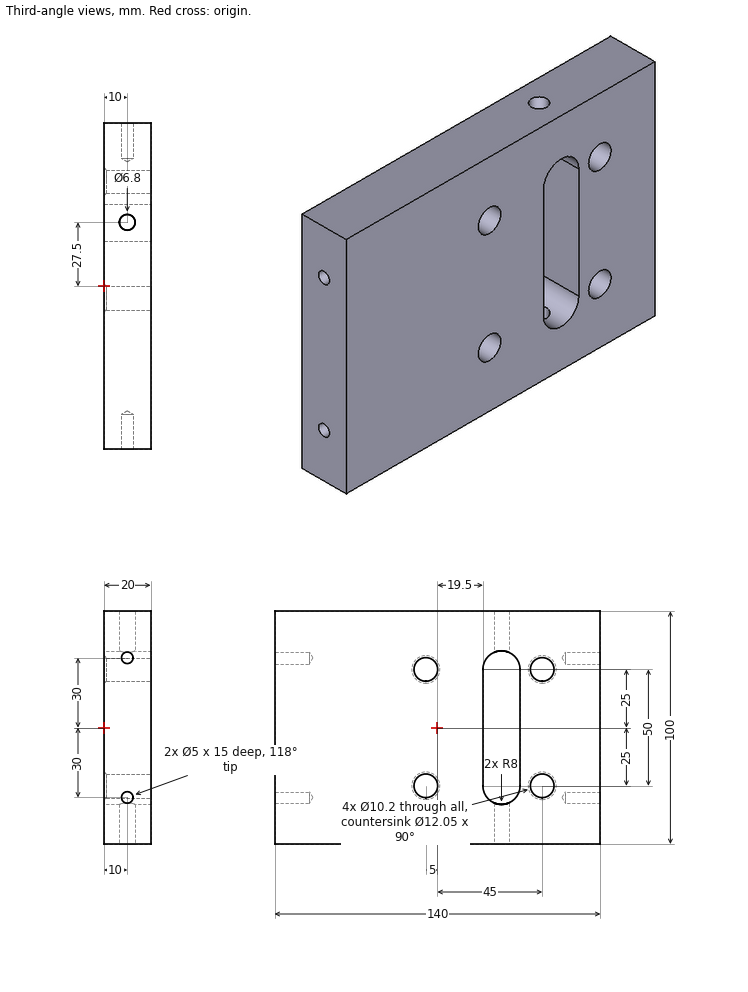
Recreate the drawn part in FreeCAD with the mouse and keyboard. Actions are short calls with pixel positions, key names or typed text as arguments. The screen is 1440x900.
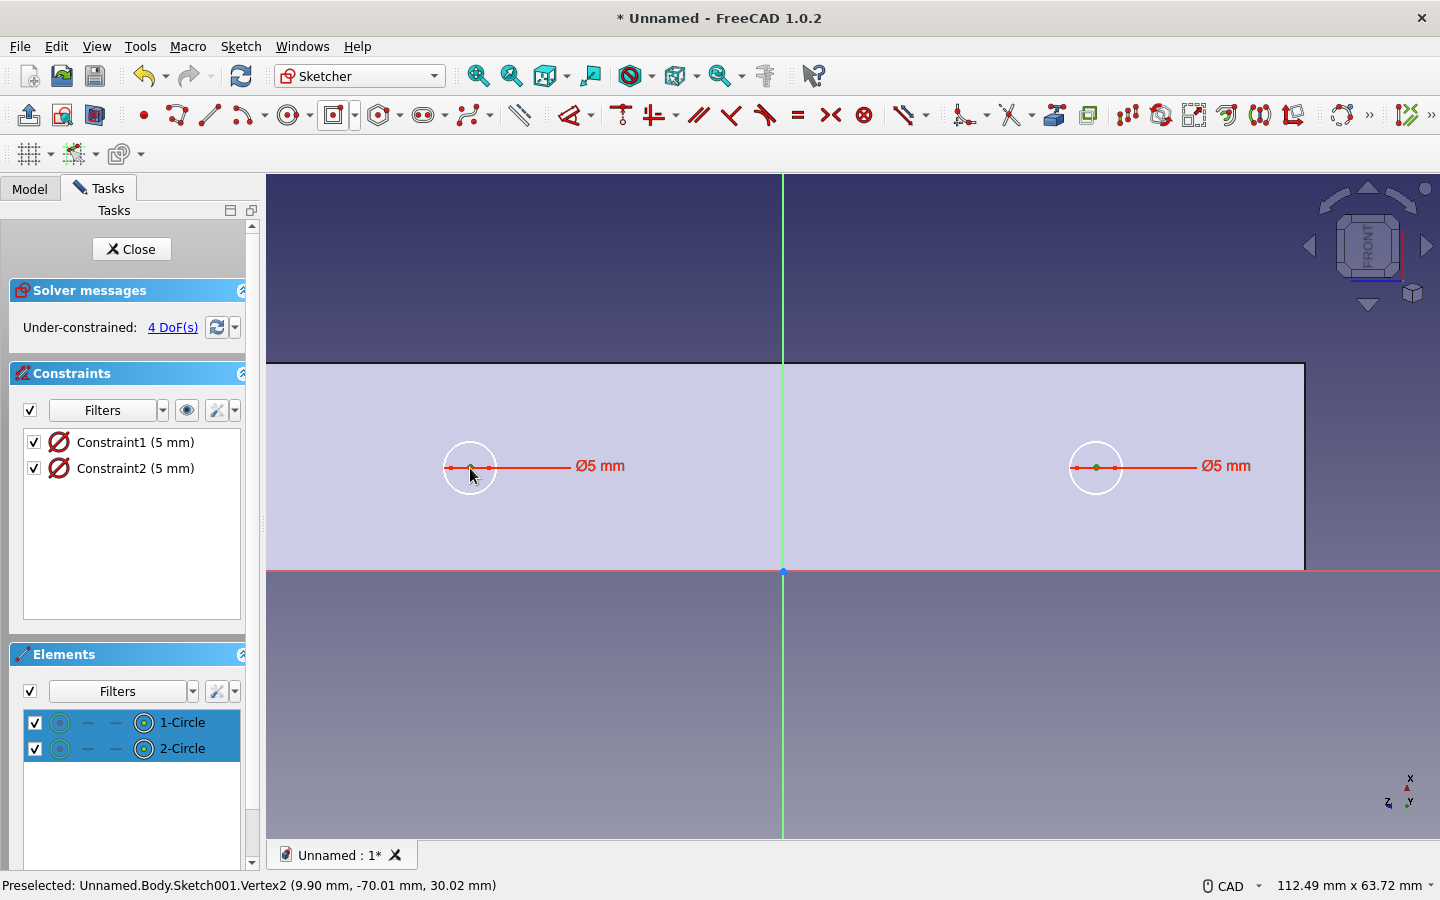
key(h)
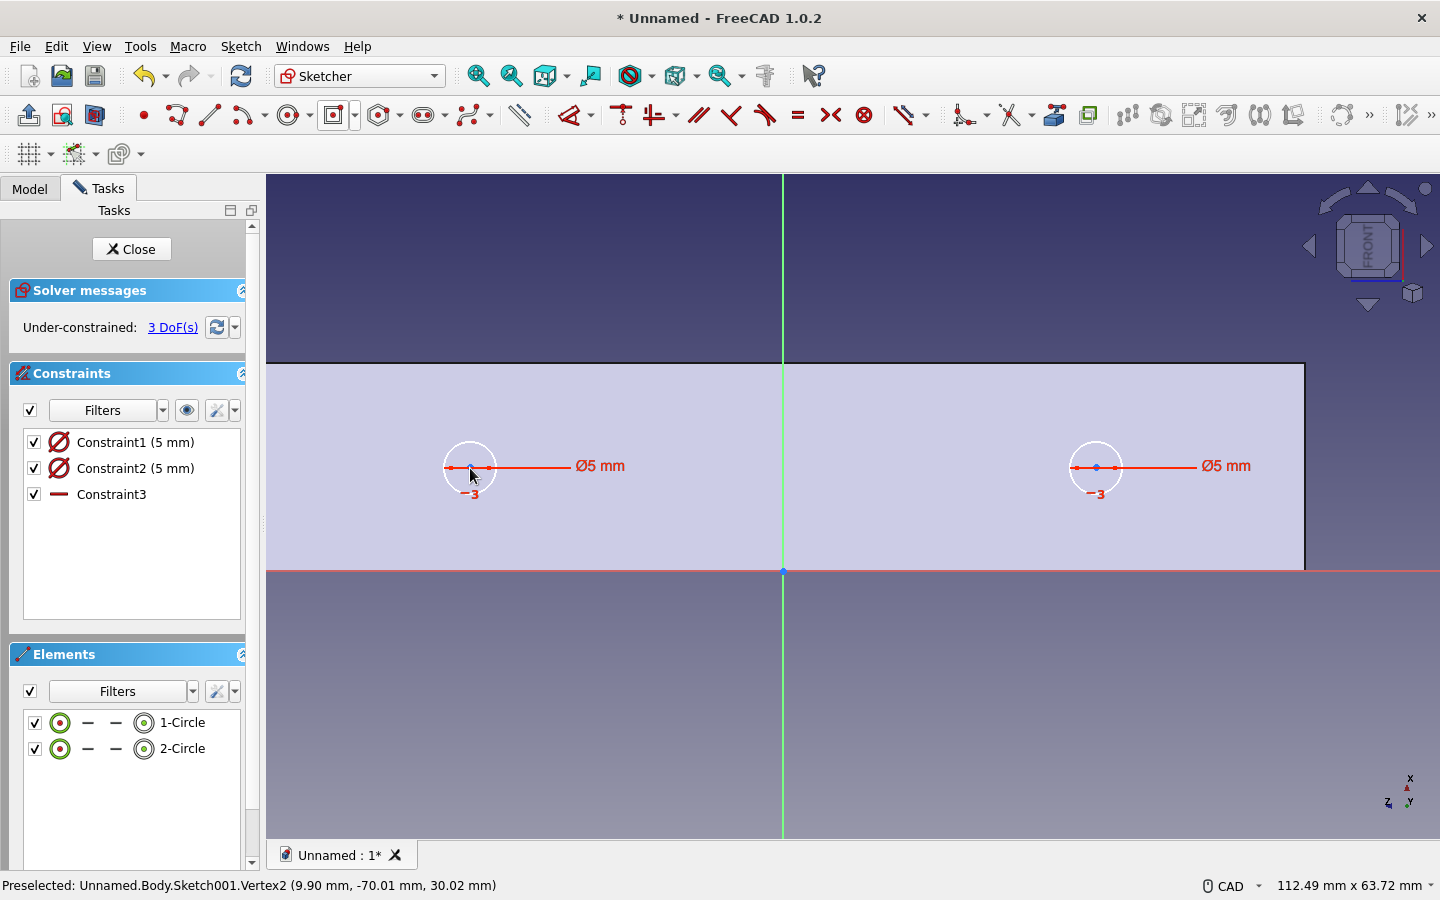
click(568, 116)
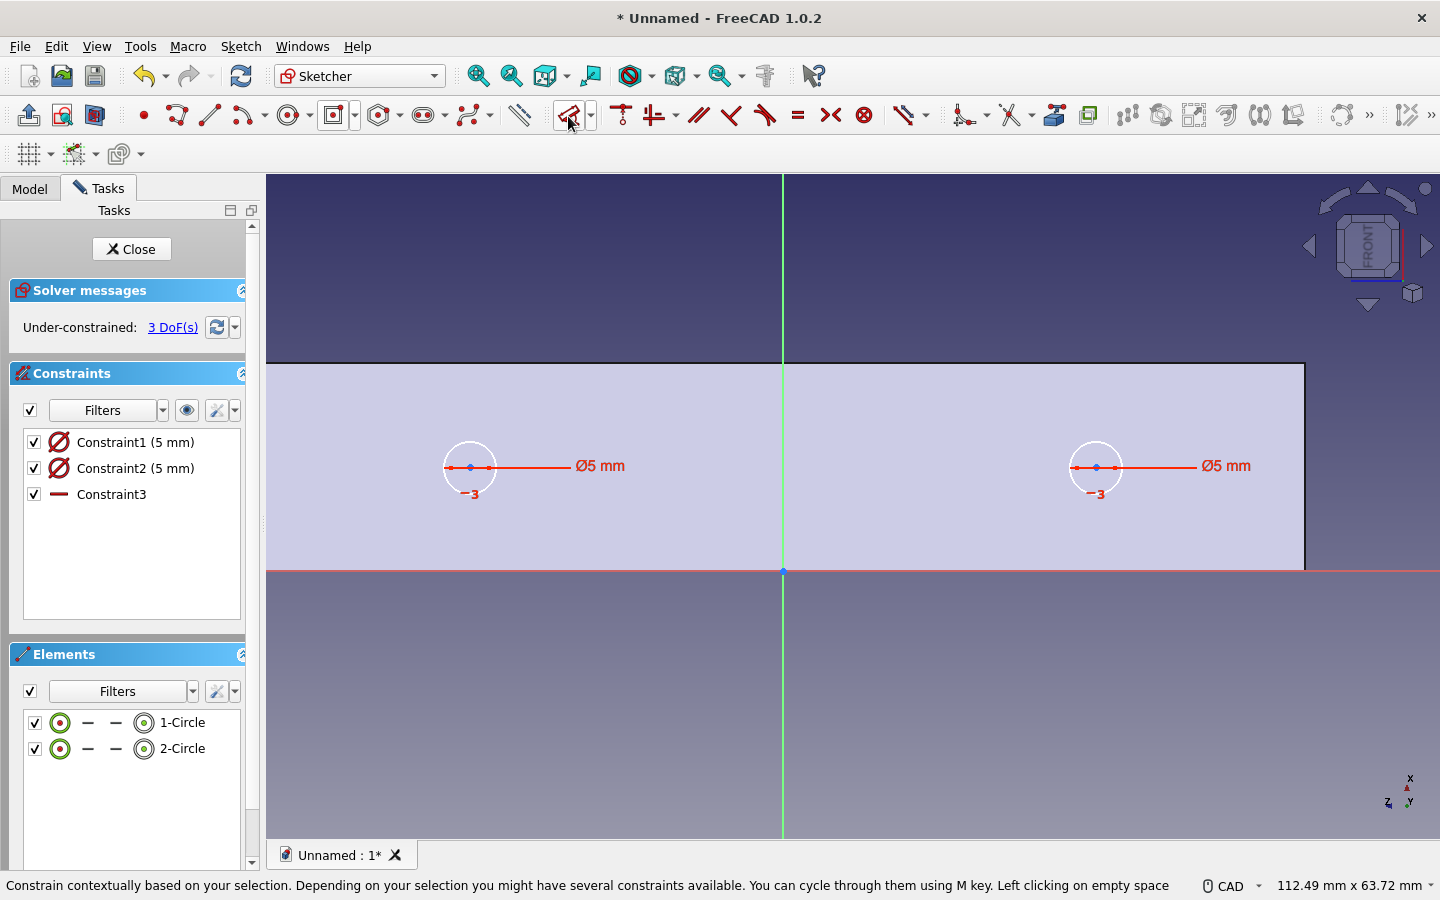
click(1096, 468)
click(940, 605)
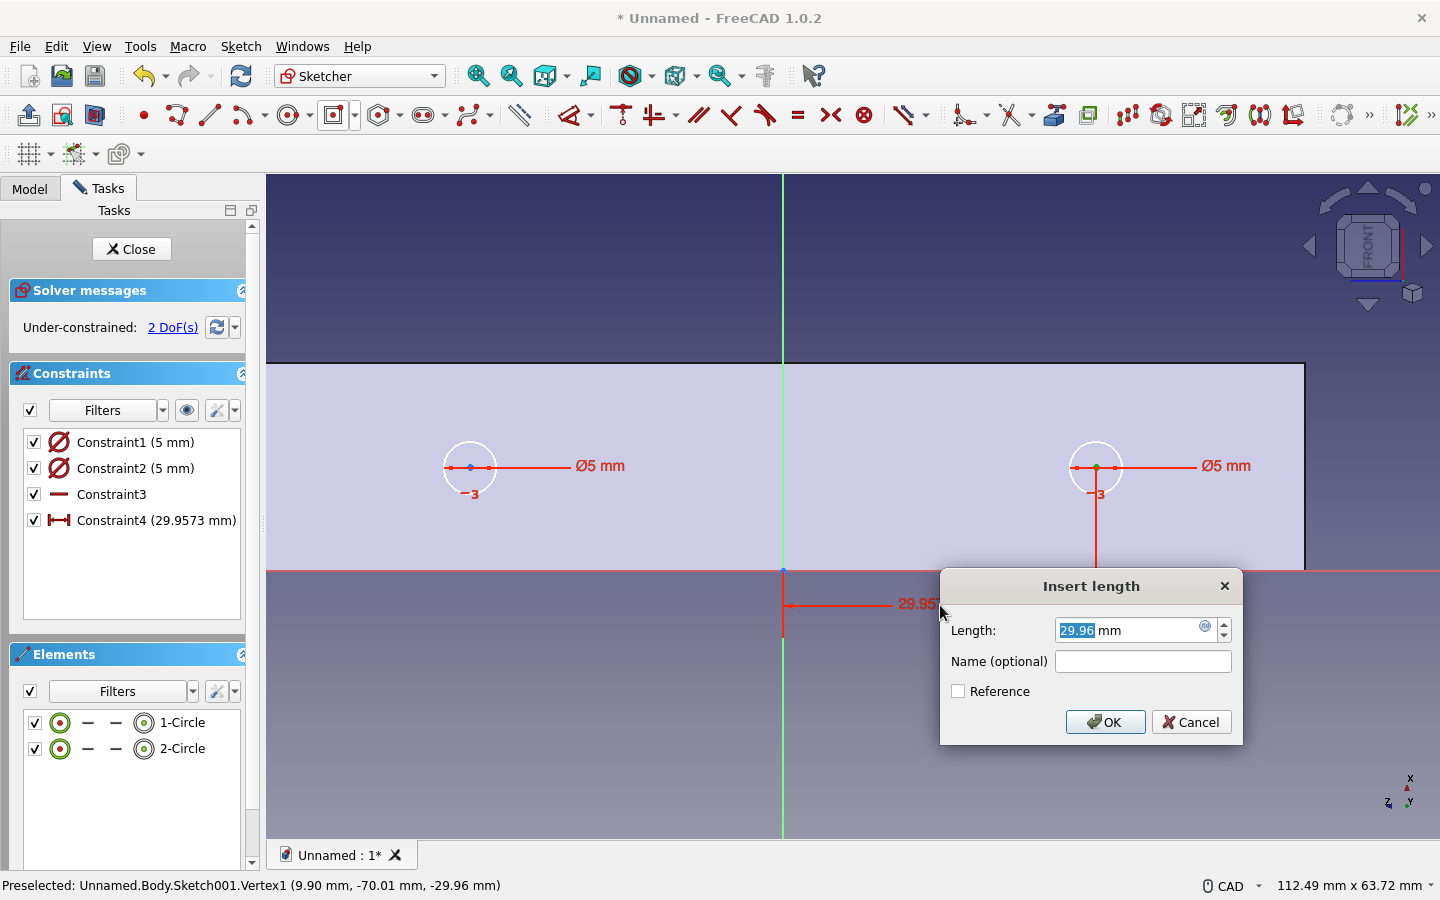
text(30)
key(Return)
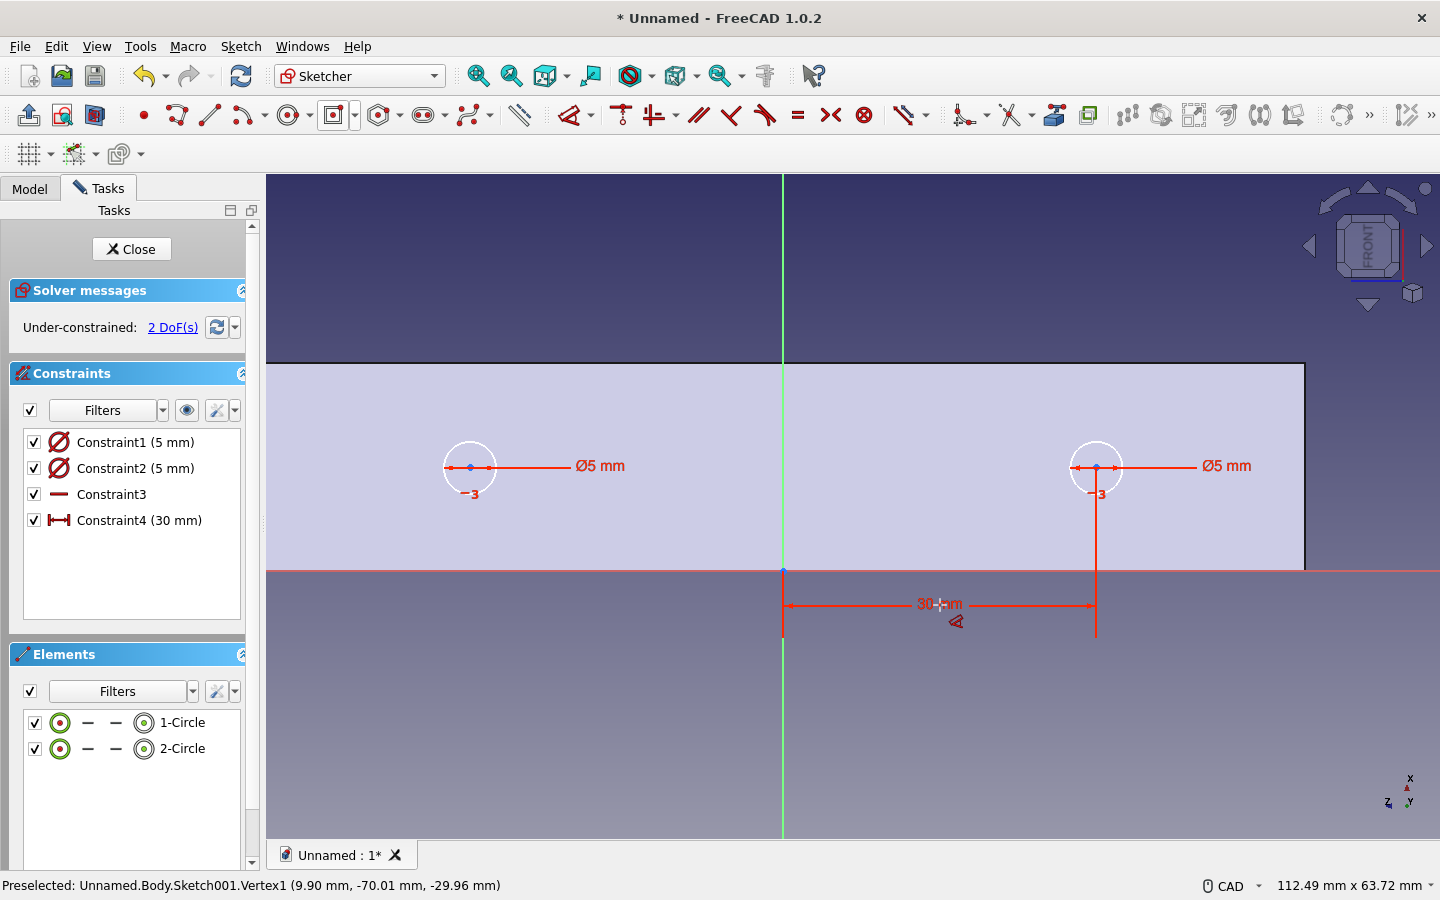
click(1096, 468)
click(1130, 520)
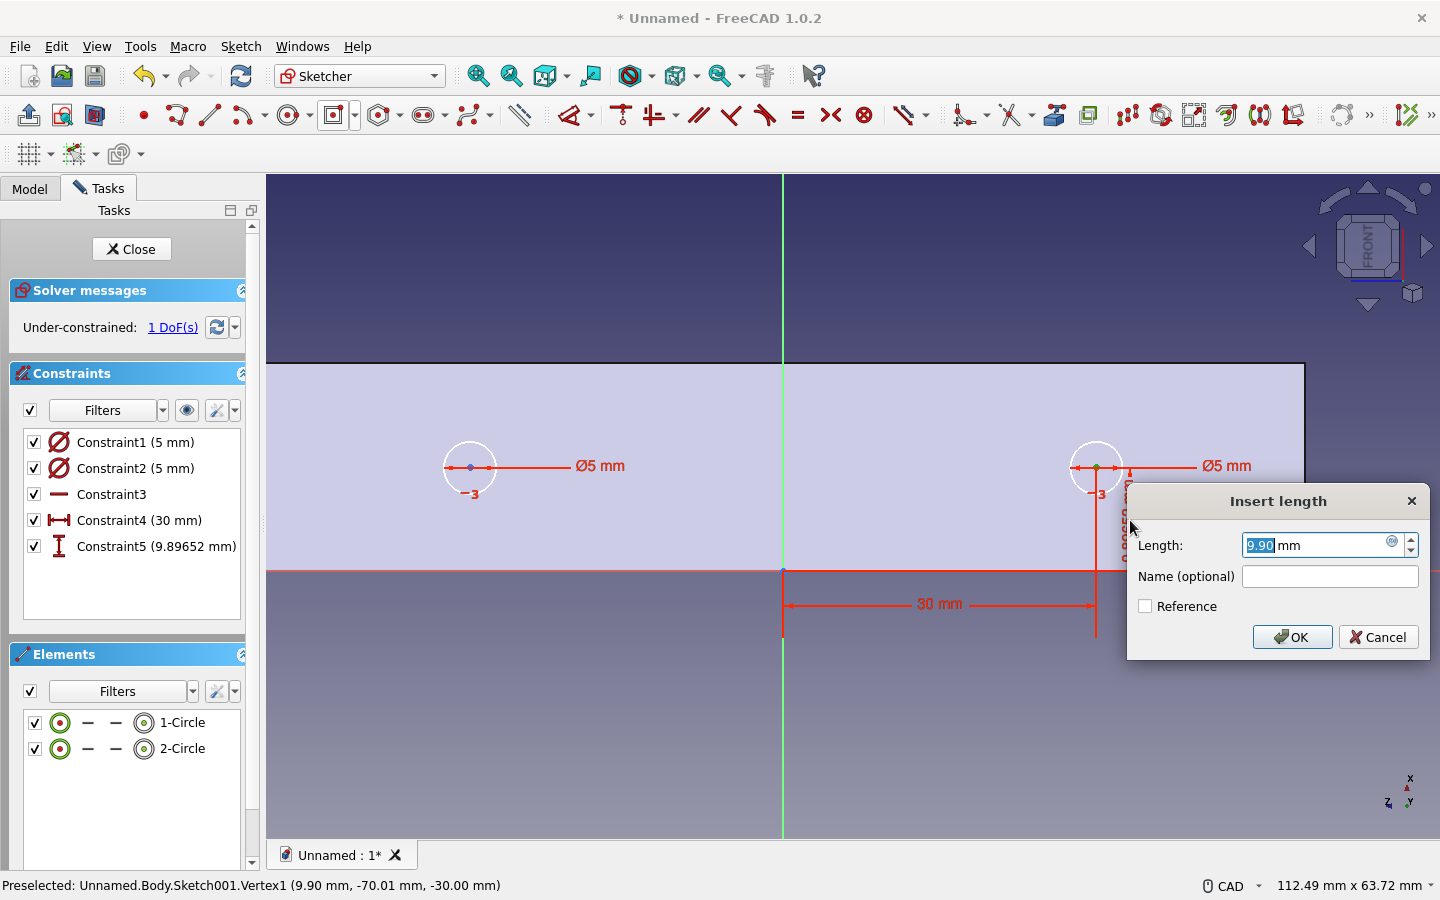
text(10)
key(Return)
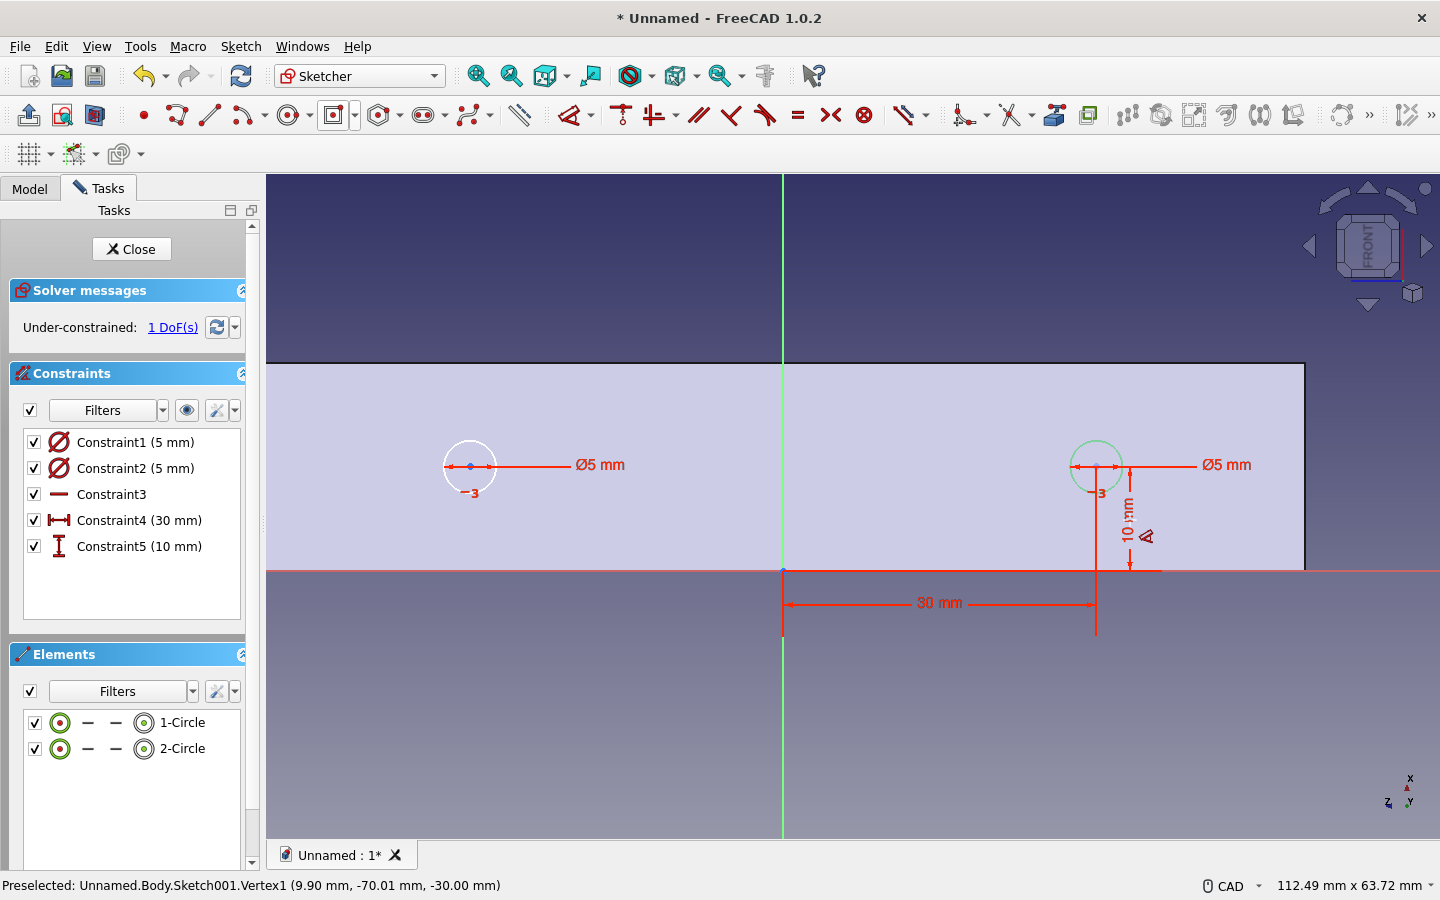
click(470, 467)
click(627, 605)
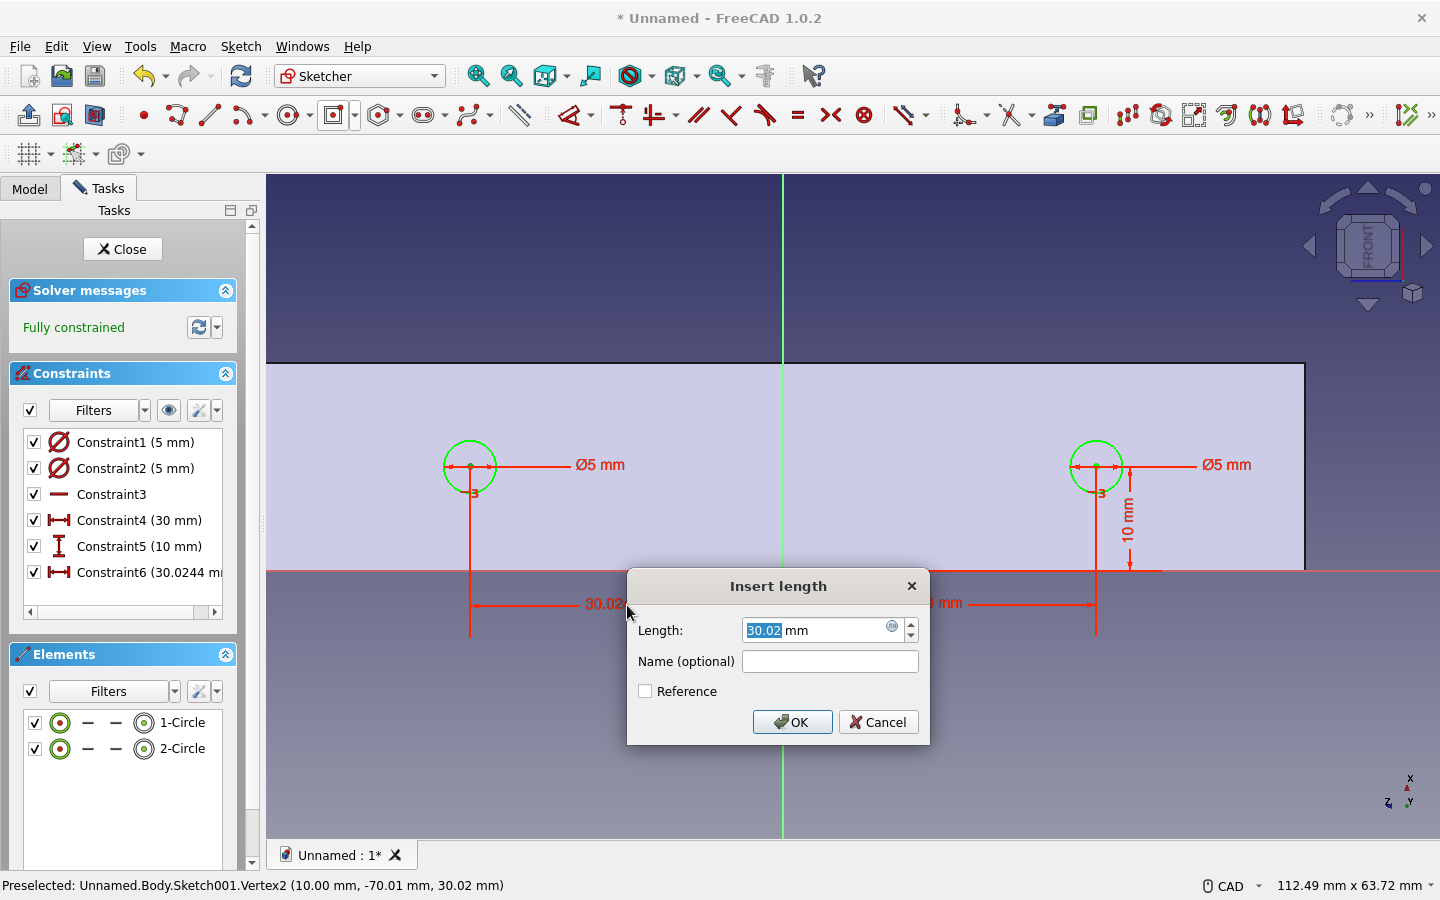
text(30)
key(Return)
key(Escape)